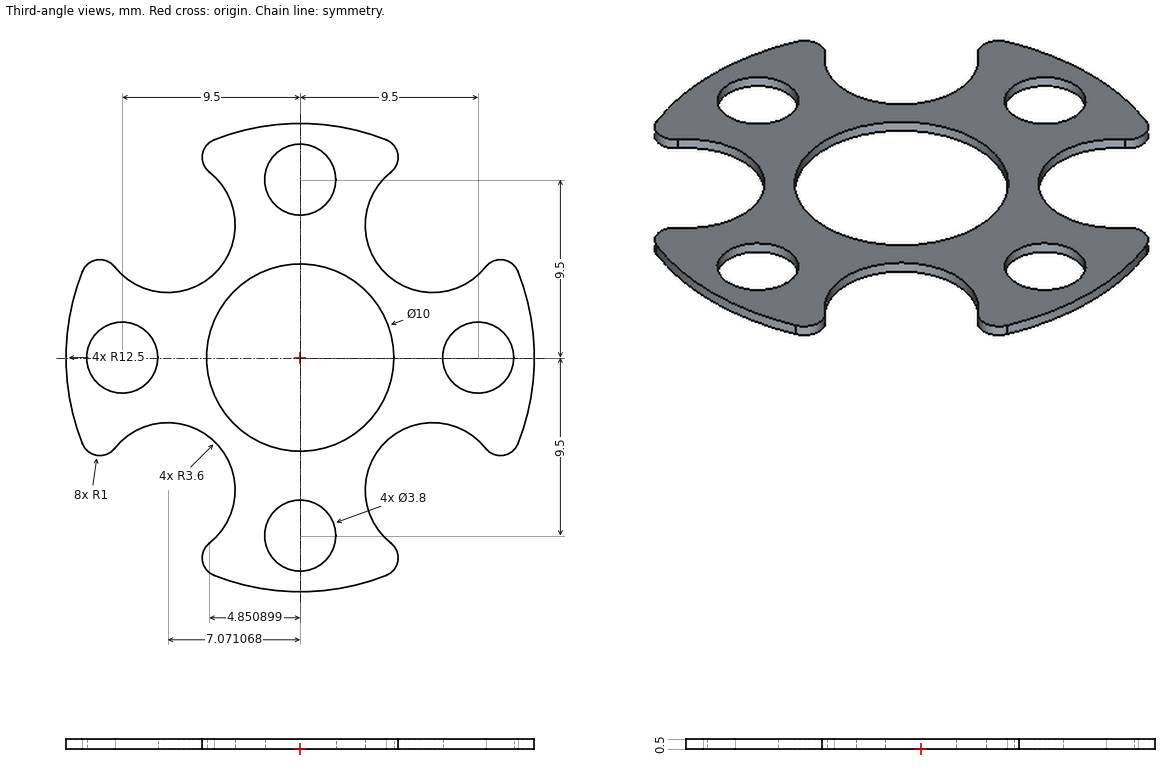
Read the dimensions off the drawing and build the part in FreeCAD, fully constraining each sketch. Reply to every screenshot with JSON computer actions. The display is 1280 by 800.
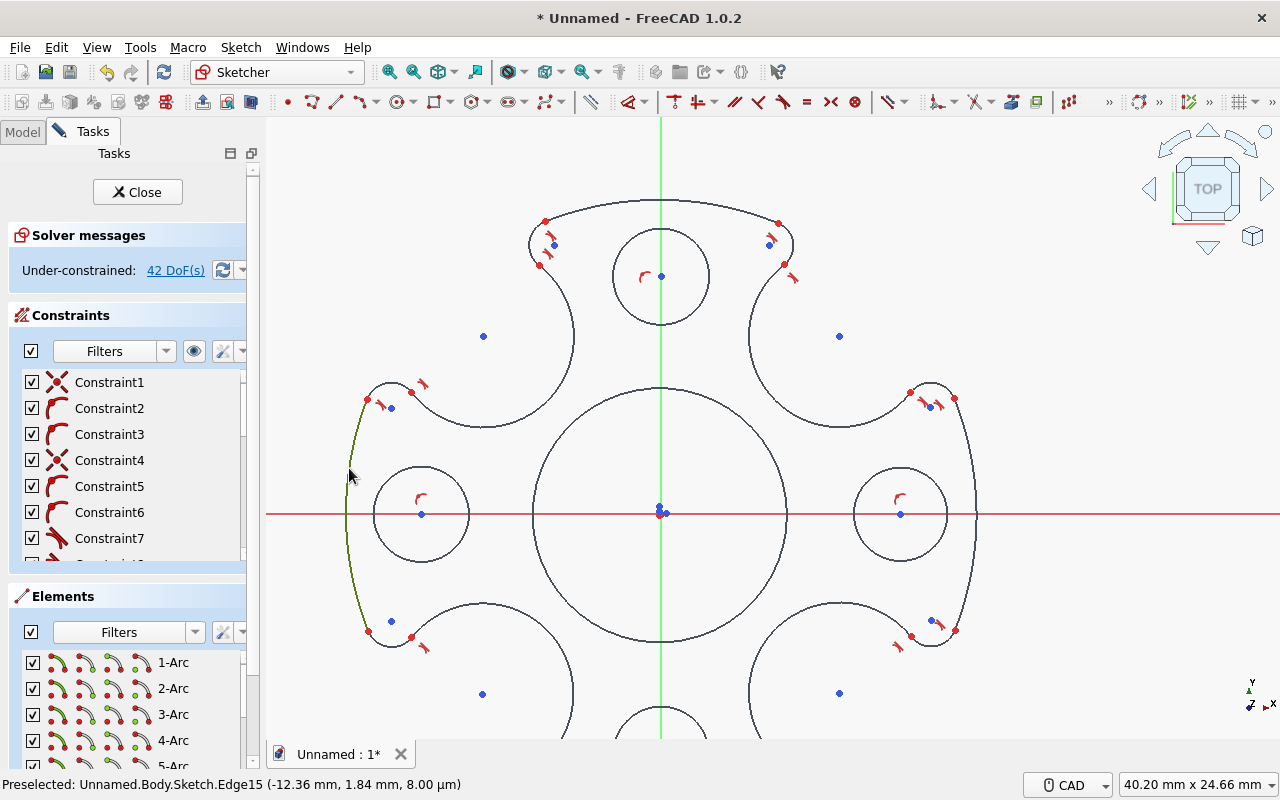
{"action": "left_click", "coordinate": [378, 643]}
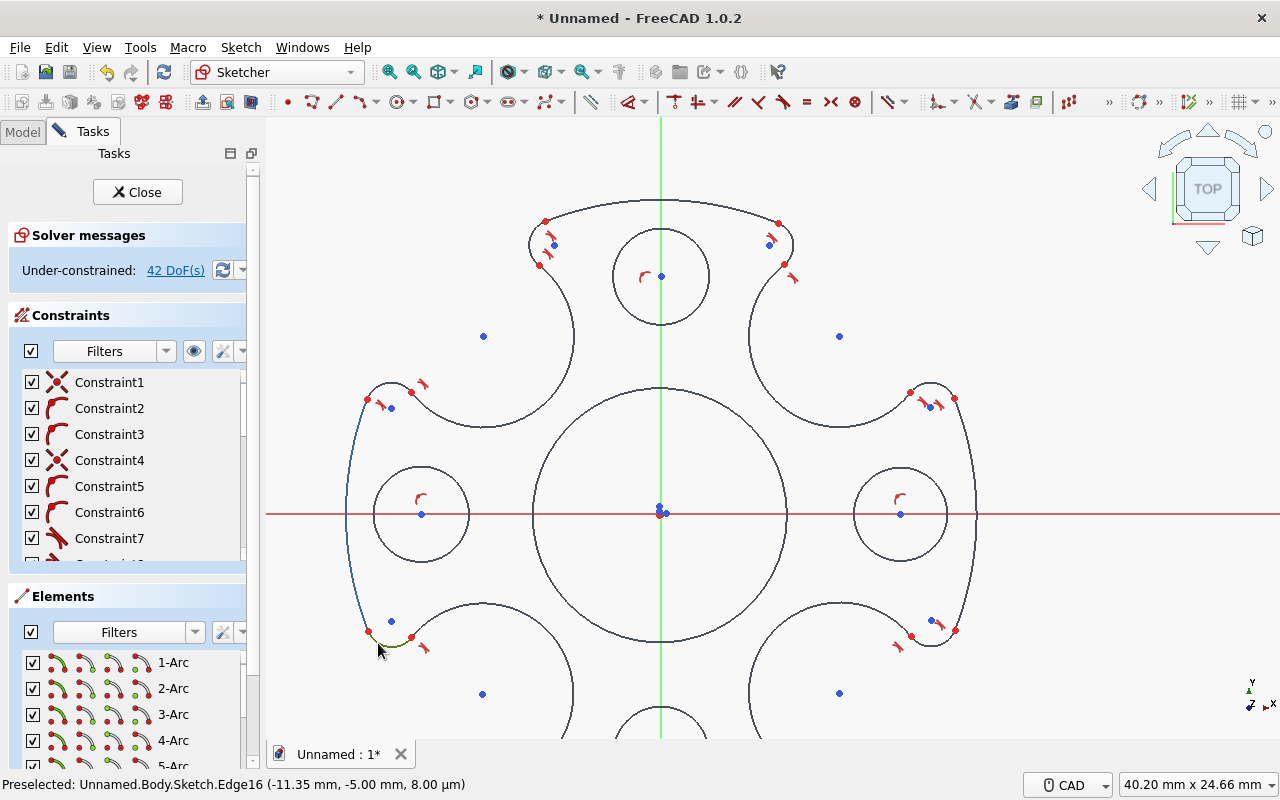
{"action": "key", "text": "t"}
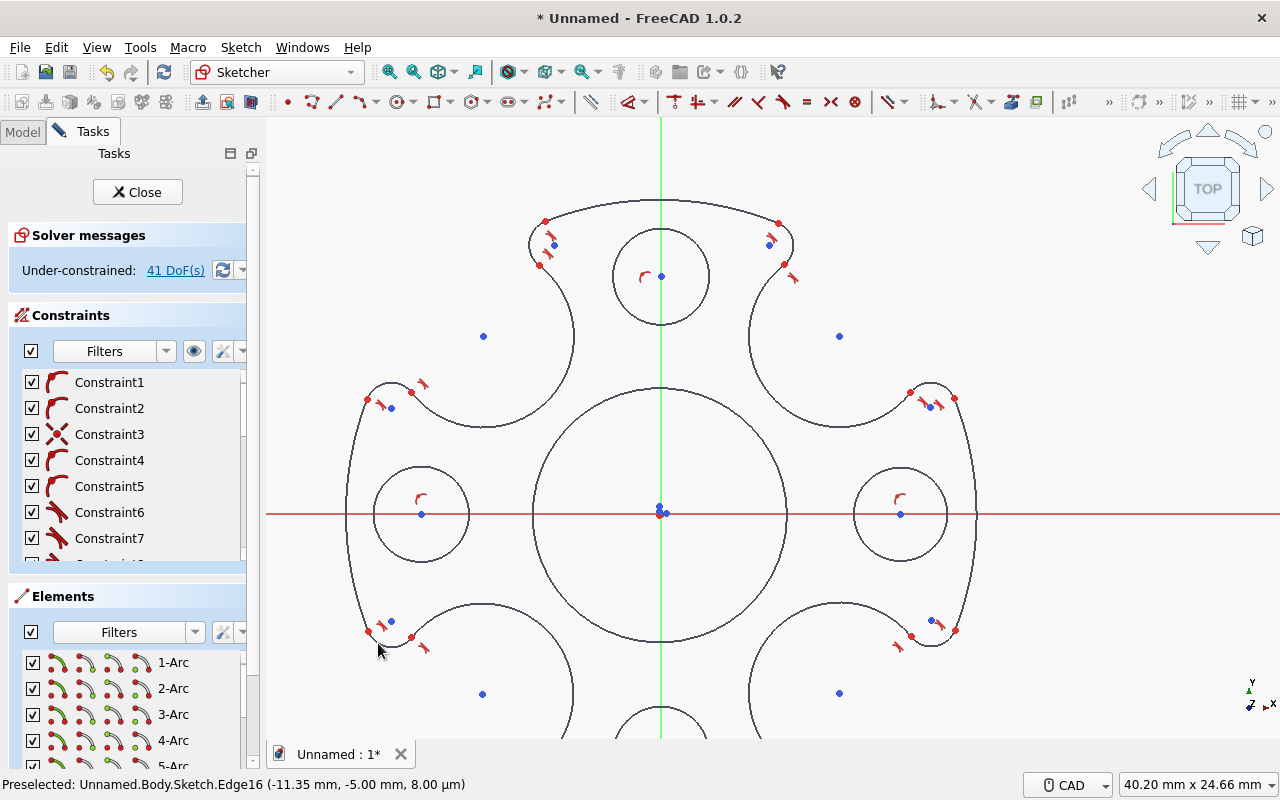
{"action": "left_click", "coordinate": [749, 425]}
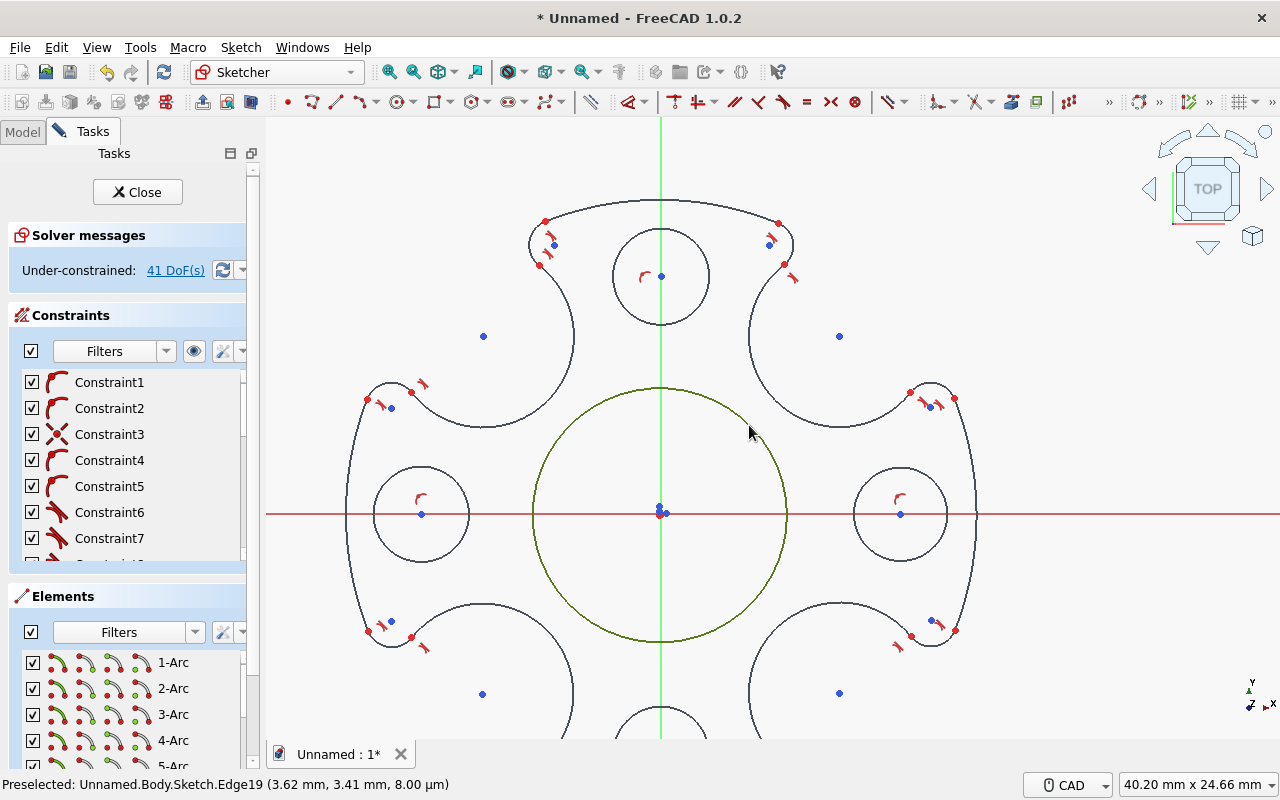
{"action": "scroll", "coordinate": [793, 252], "scroll_direction": "down", "scroll_amount": 2}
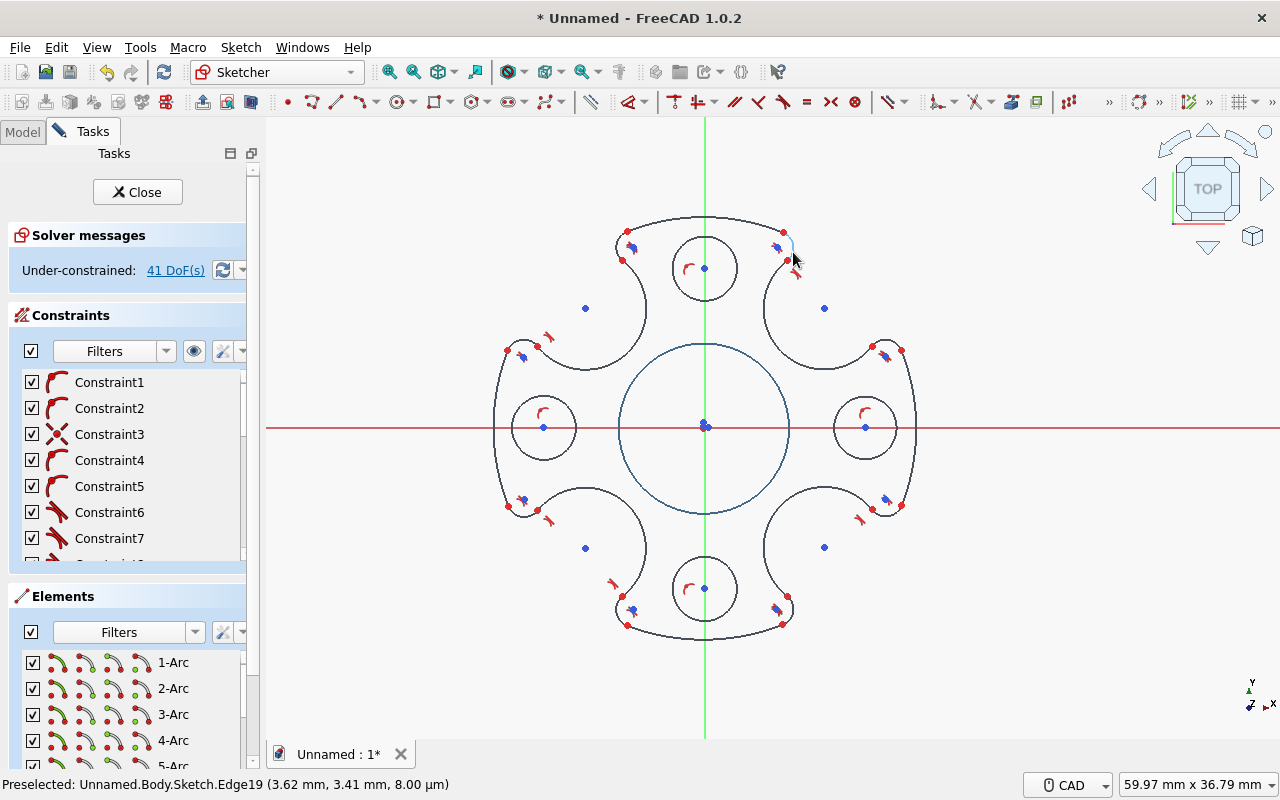
{"action": "left_click", "coordinate": [674, 638]}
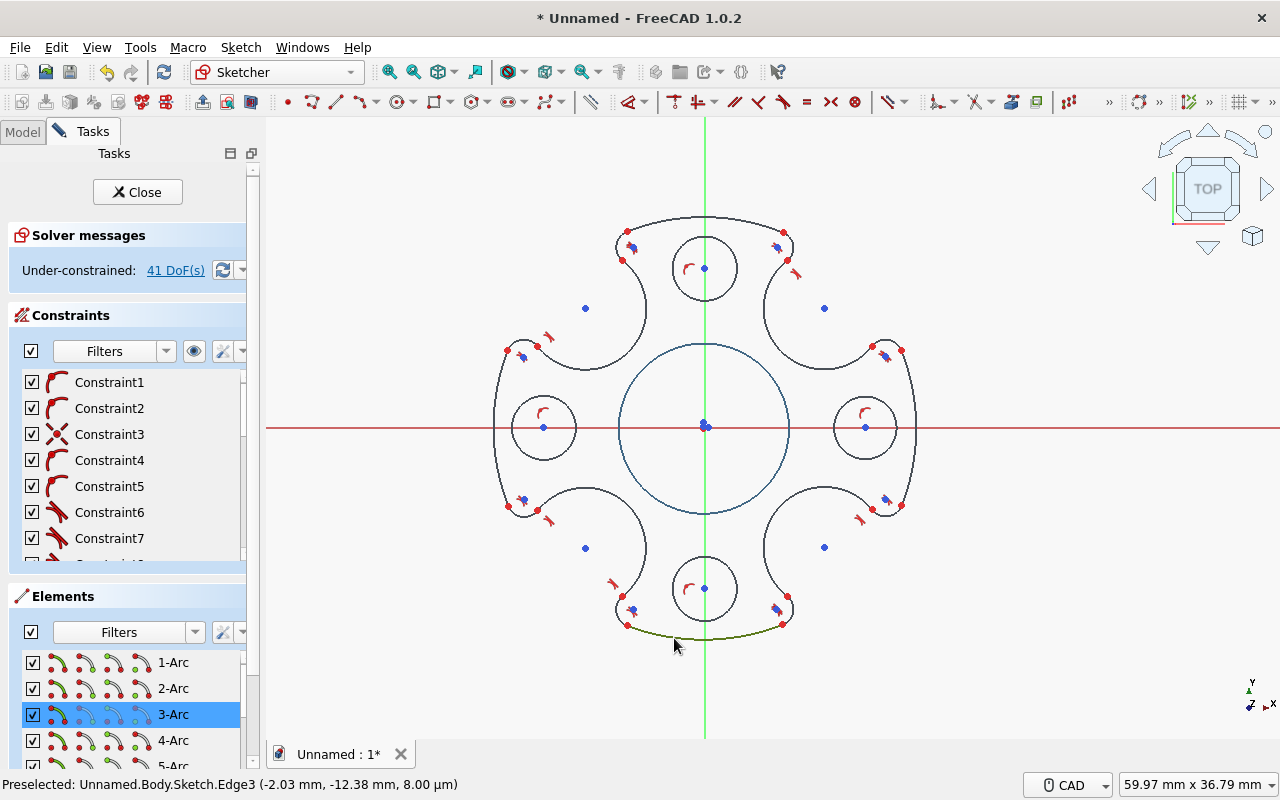
{"action": "left_click", "coordinate": [674, 102]}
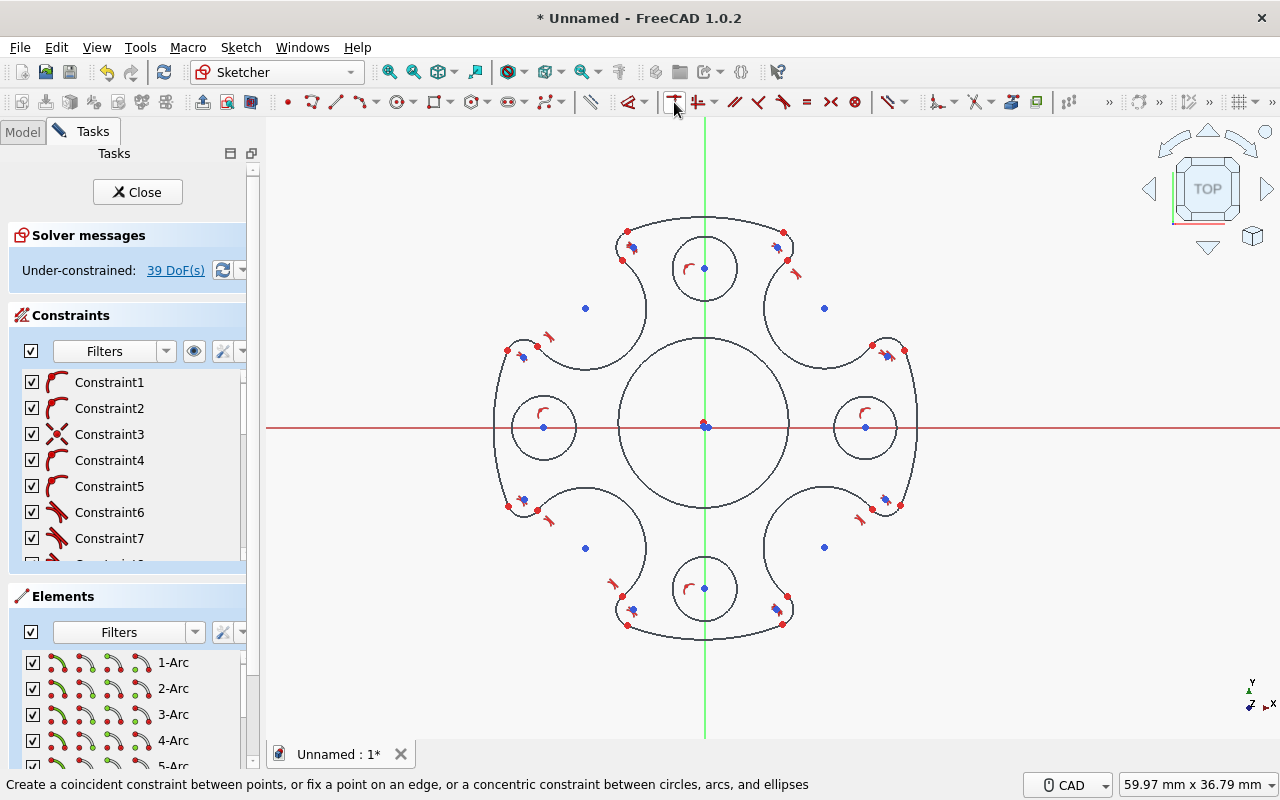
{"action": "left_click", "coordinate": [764, 362]}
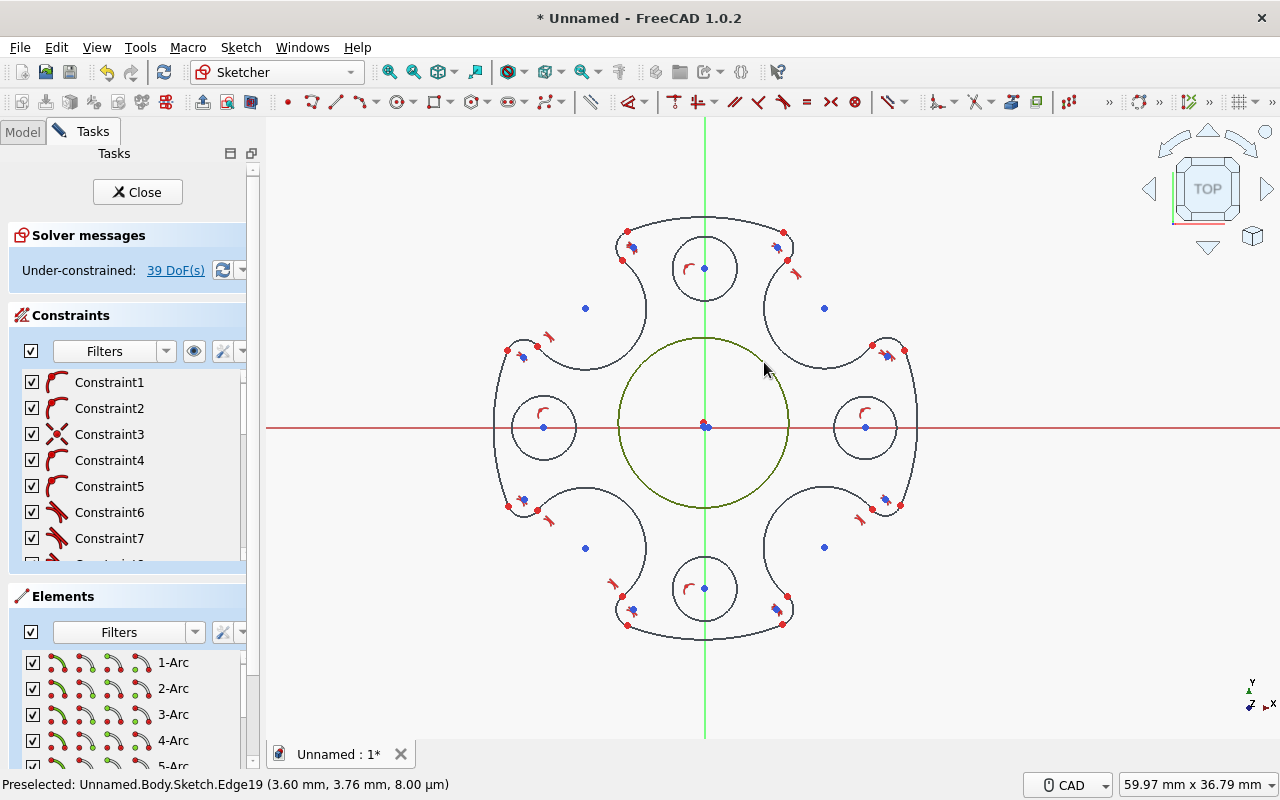
{"action": "left_click", "coordinate": [737, 220]}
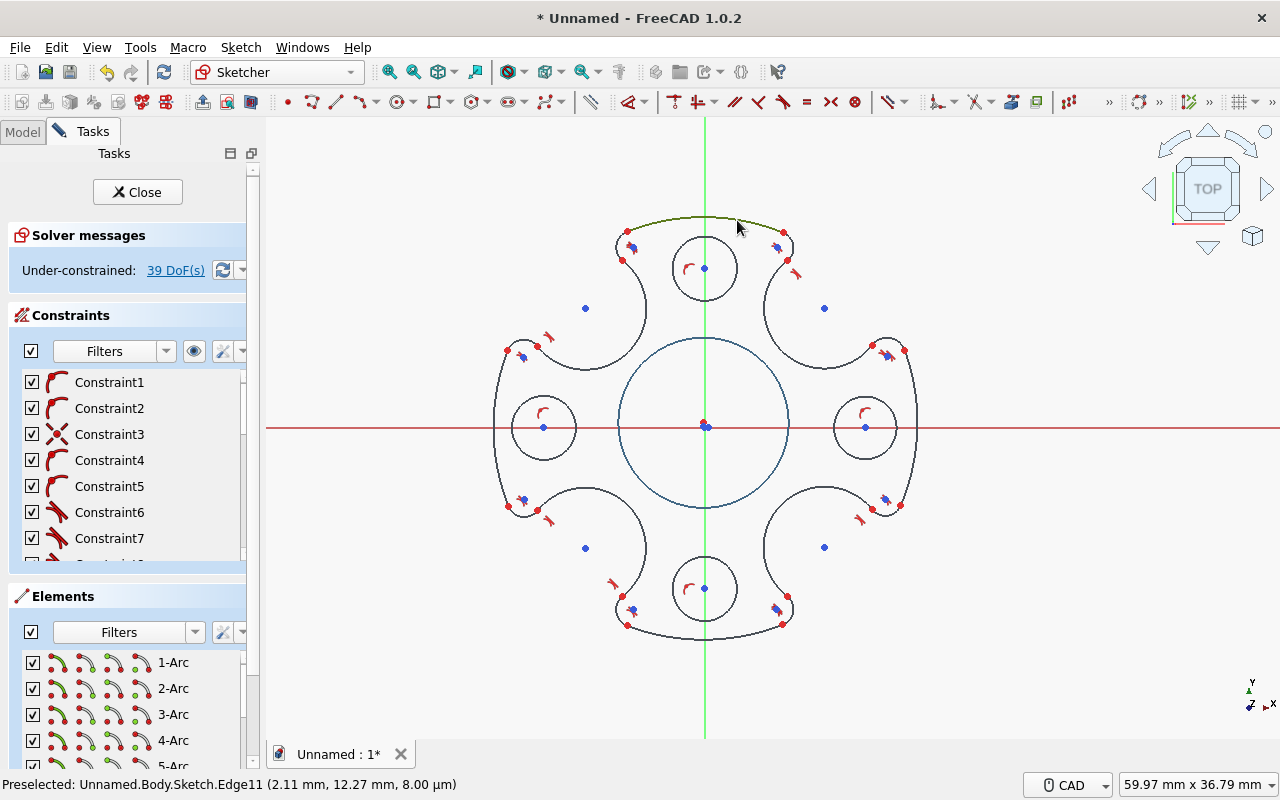
{"action": "key", "text": "c"}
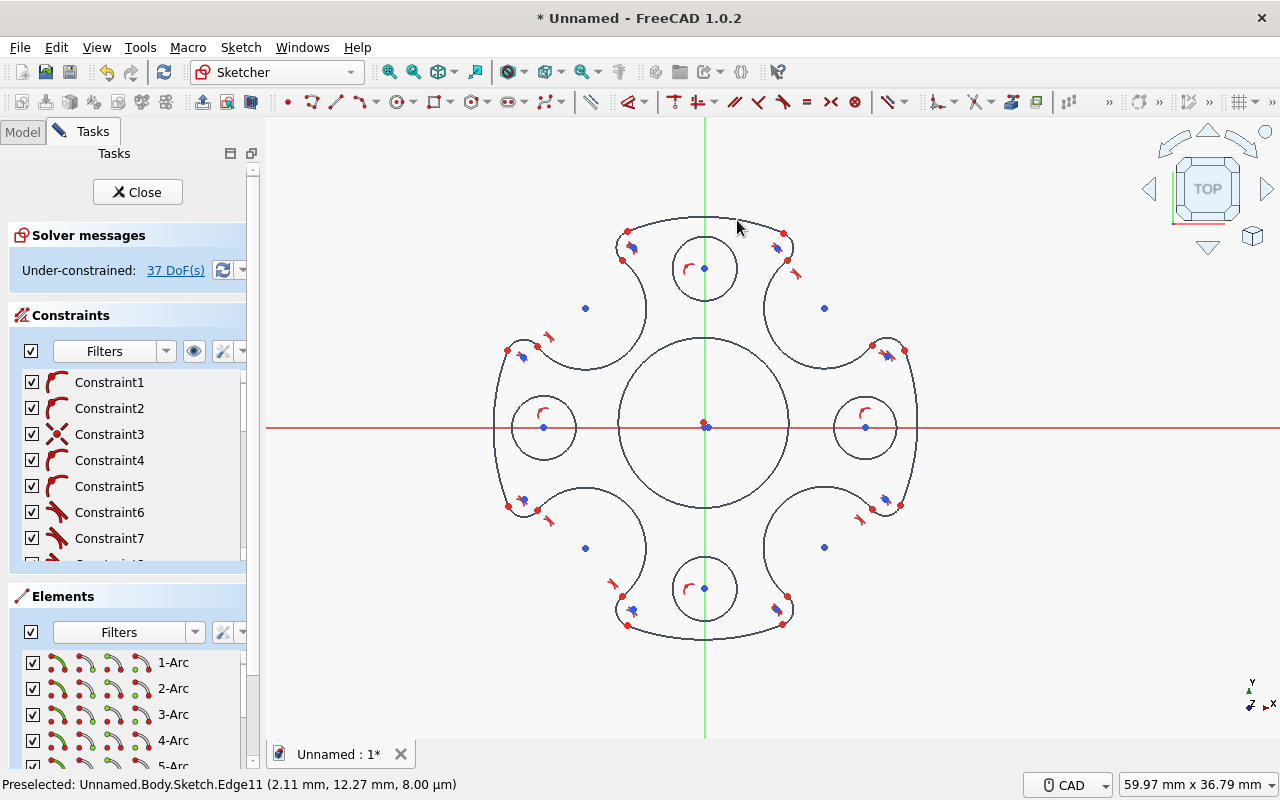
{"action": "left_click", "coordinate": [764, 362]}